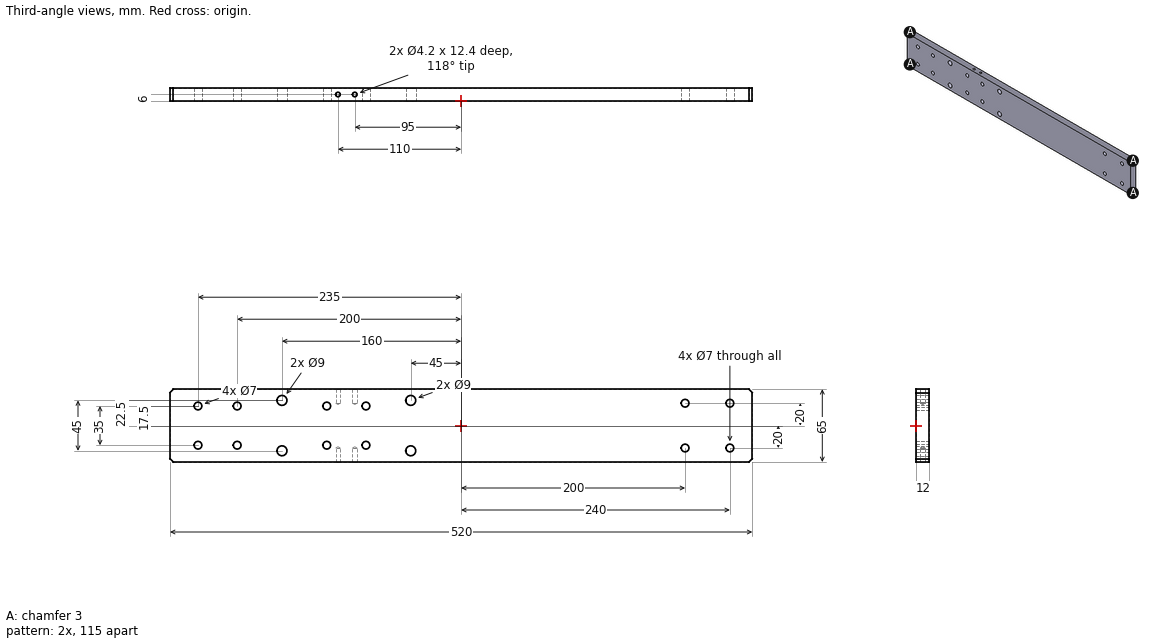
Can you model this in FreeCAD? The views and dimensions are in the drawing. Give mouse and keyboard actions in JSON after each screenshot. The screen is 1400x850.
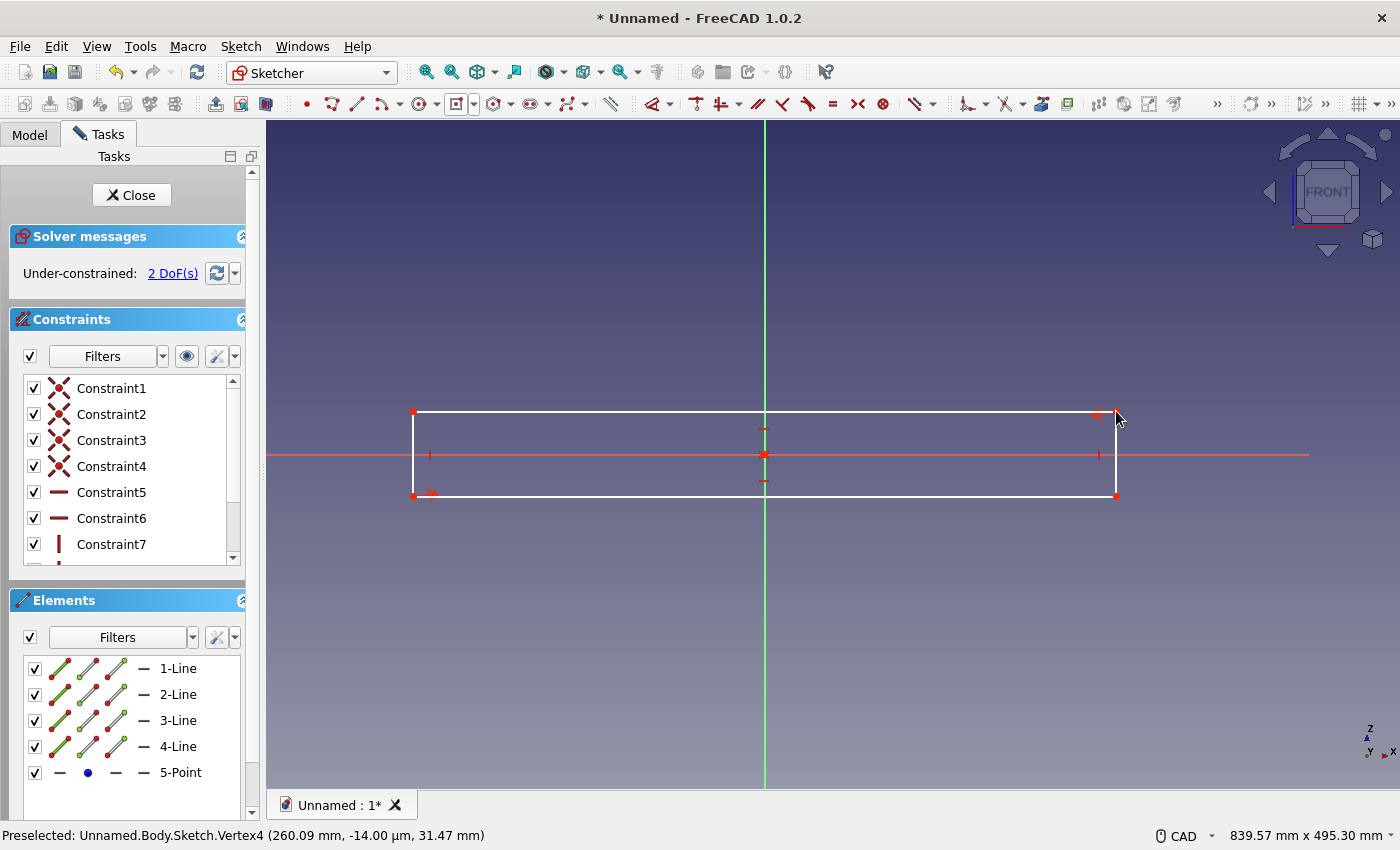
{"action": "left_click", "coordinate": [1116, 471]}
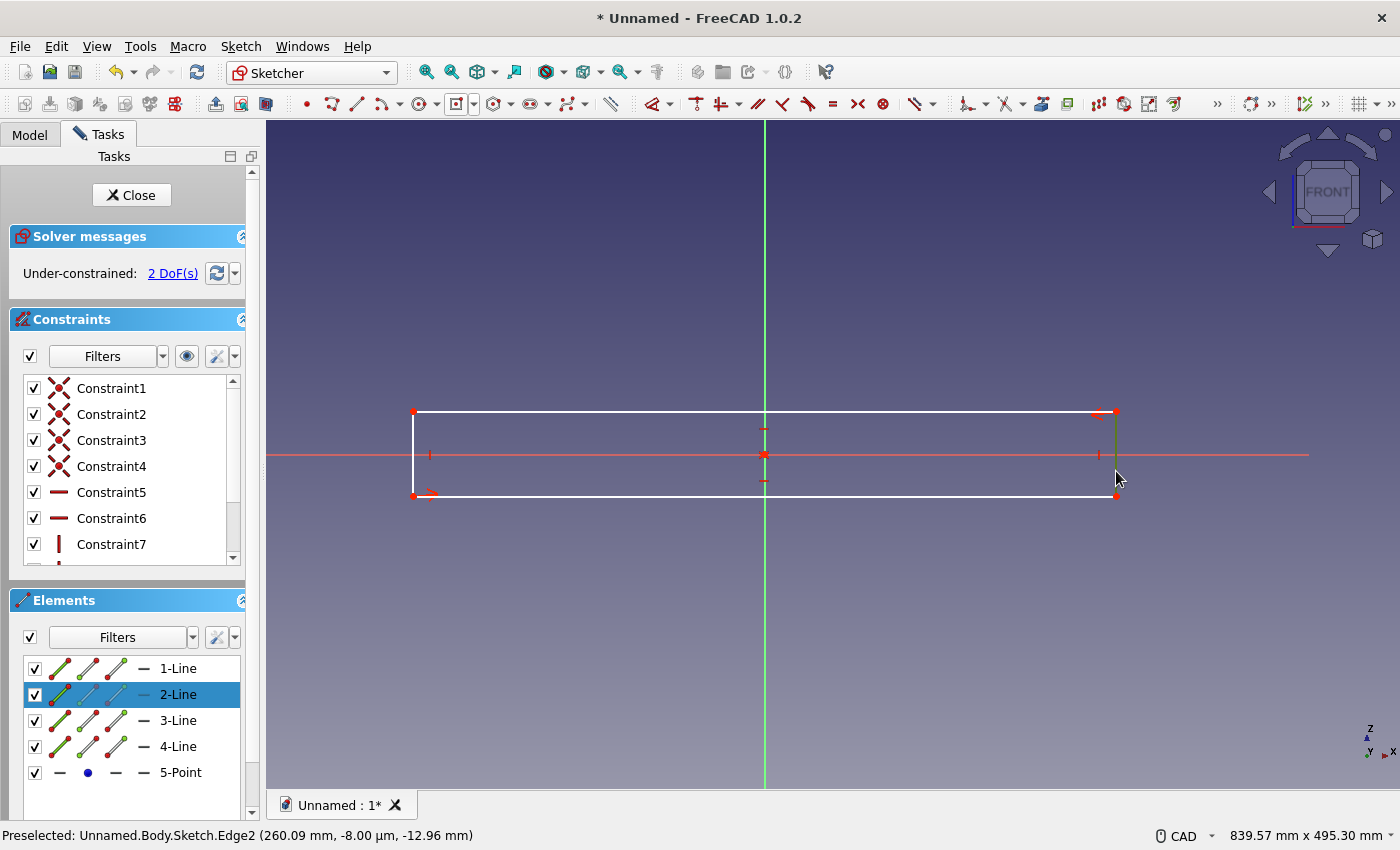
{"action": "left_click", "coordinate": [670, 104]}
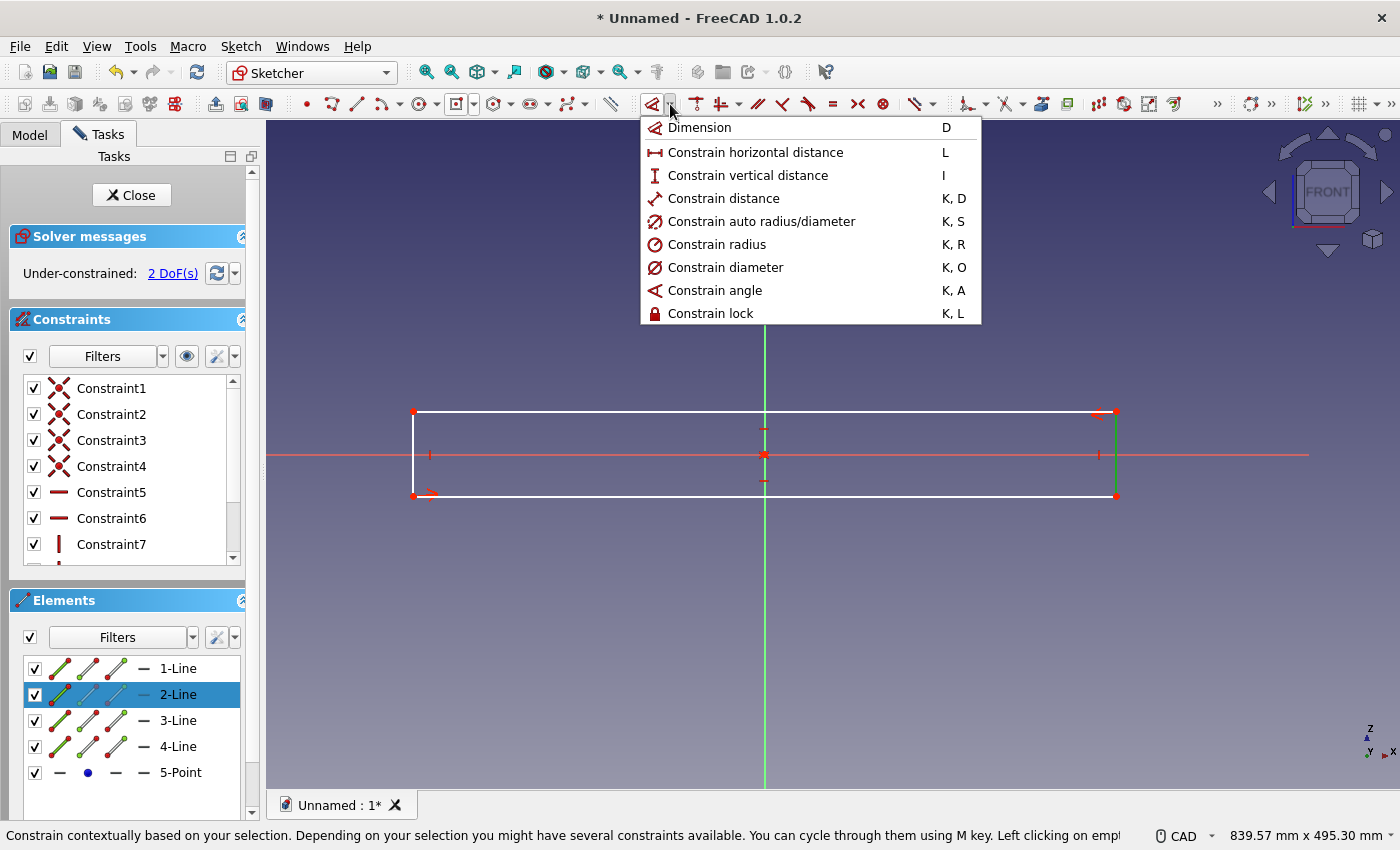
{"action": "left_click", "coordinate": [811, 176]}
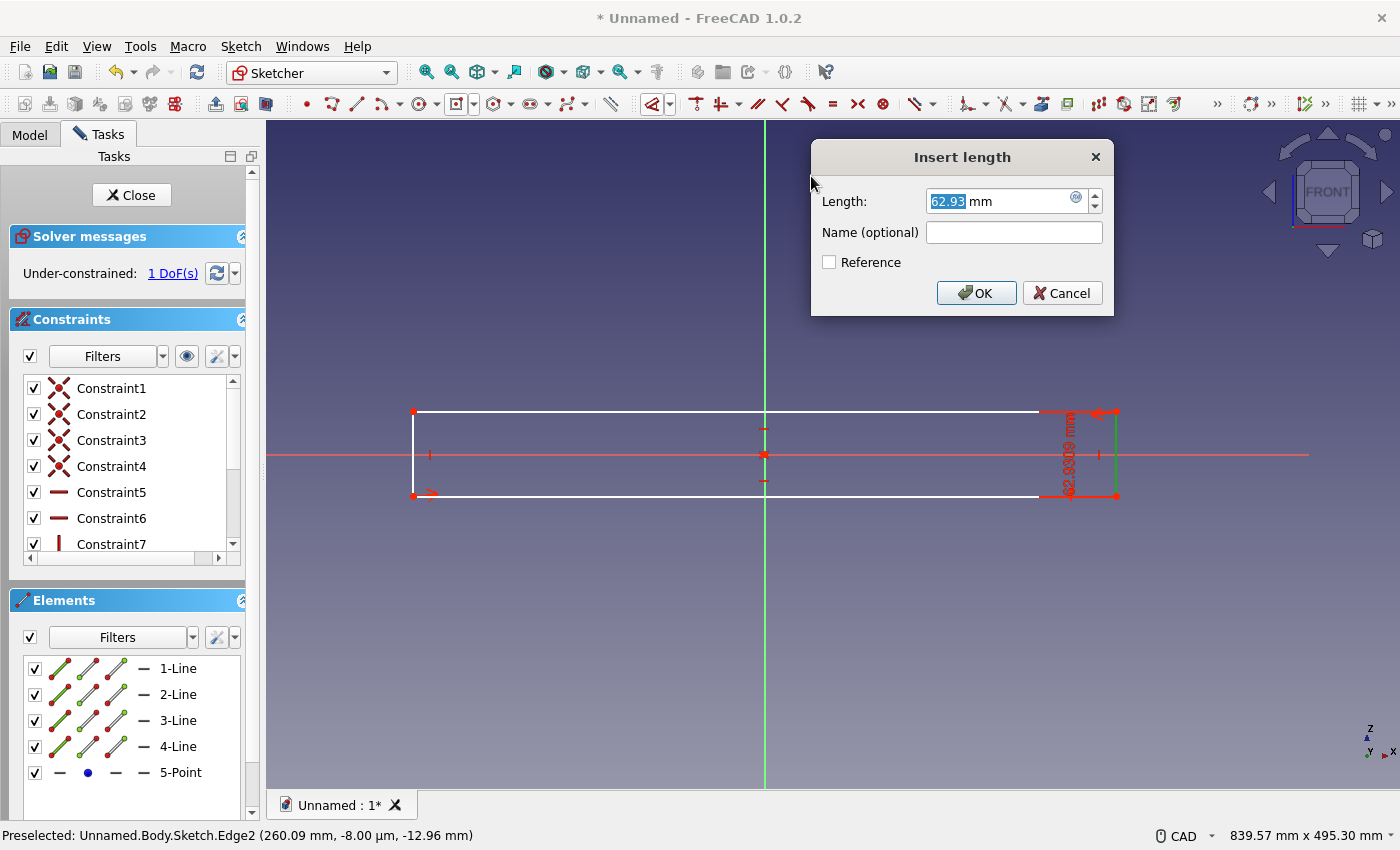
{"action": "type", "text": "65"}
{"action": "key", "text": "Return"}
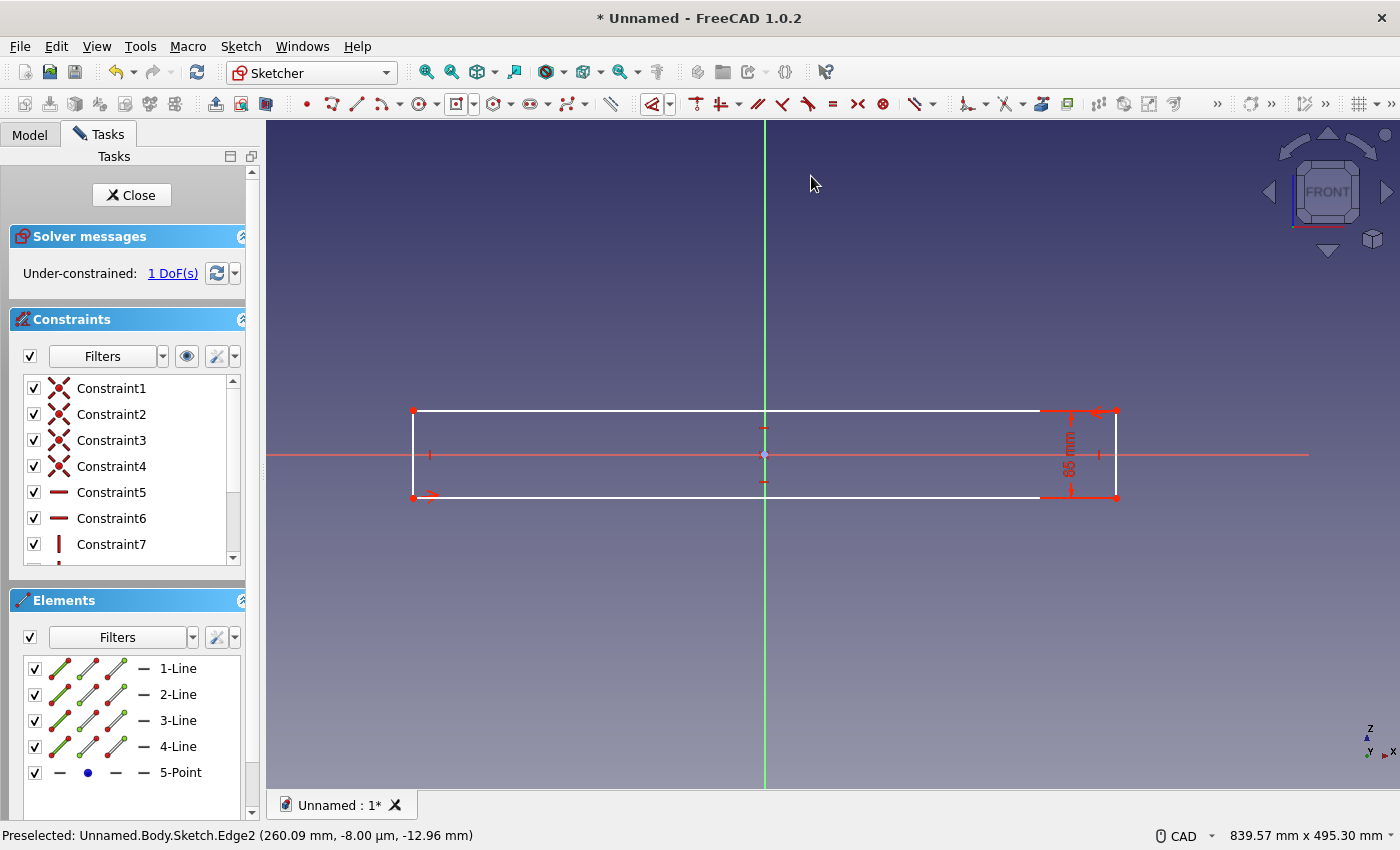
{"action": "left_click", "coordinate": [624, 498]}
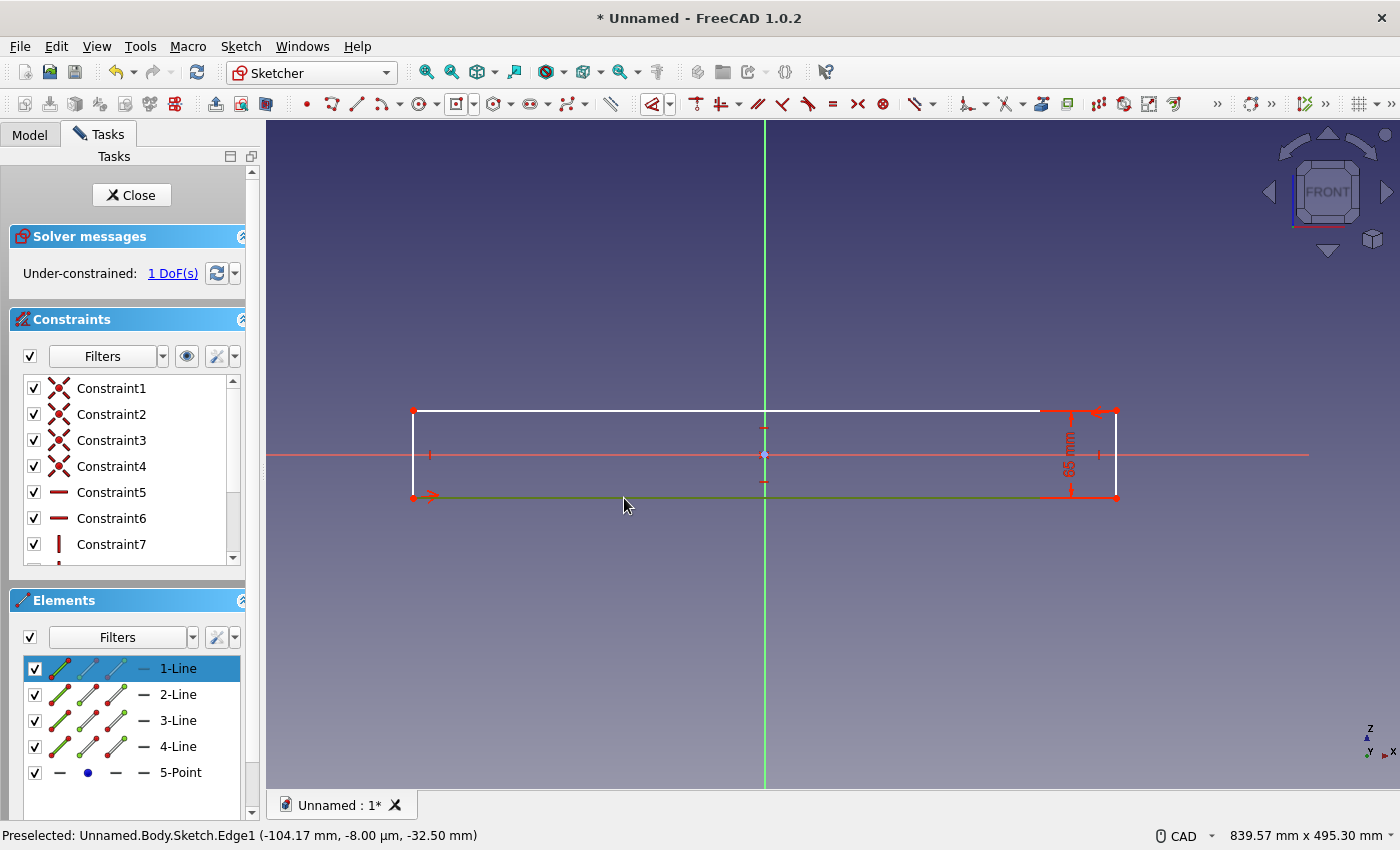
{"action": "key", "text": "l"}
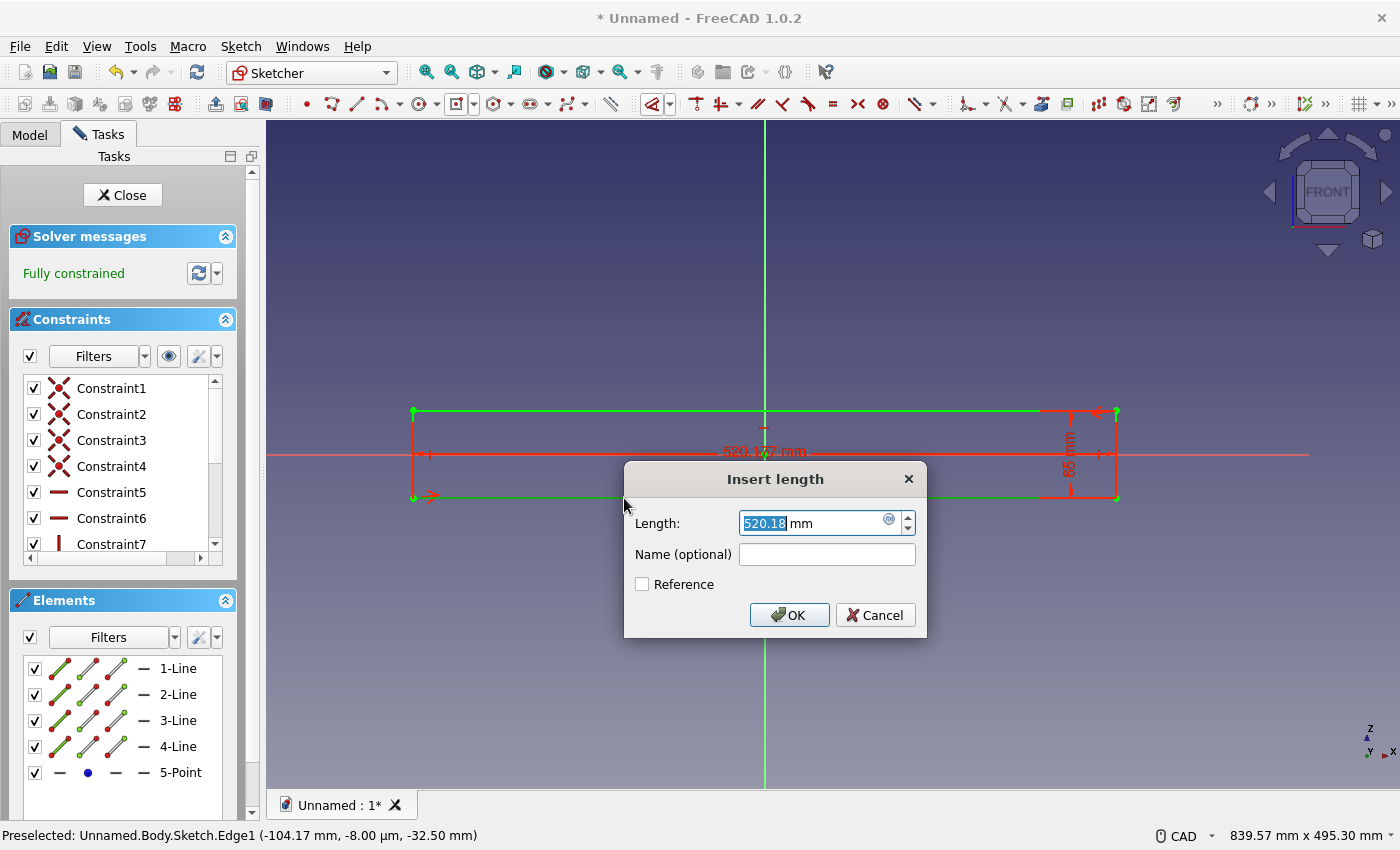
{"action": "type", "text": "520"}
{"action": "key", "text": "Return"}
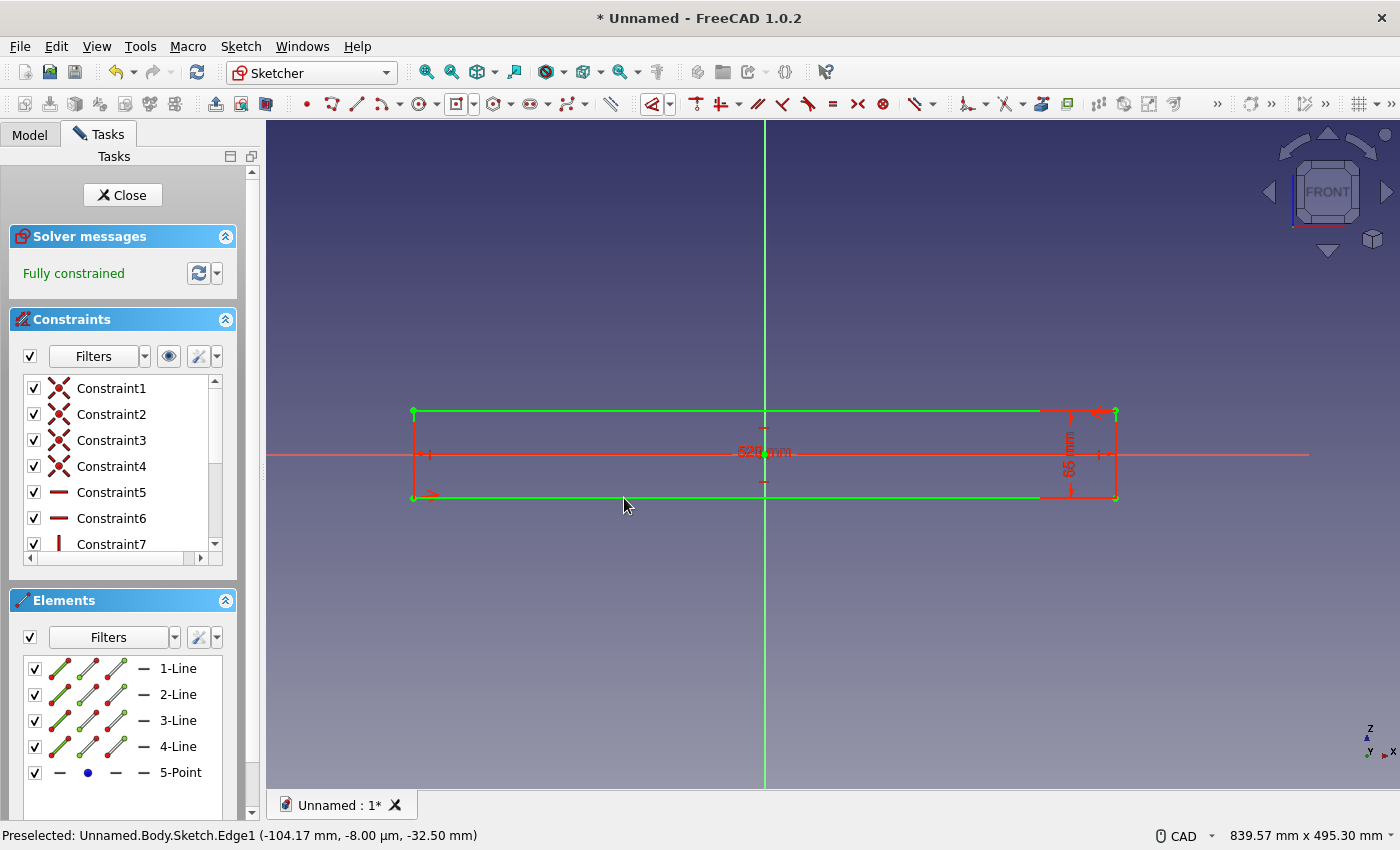
{"action": "left_click", "coordinate": [123, 195]}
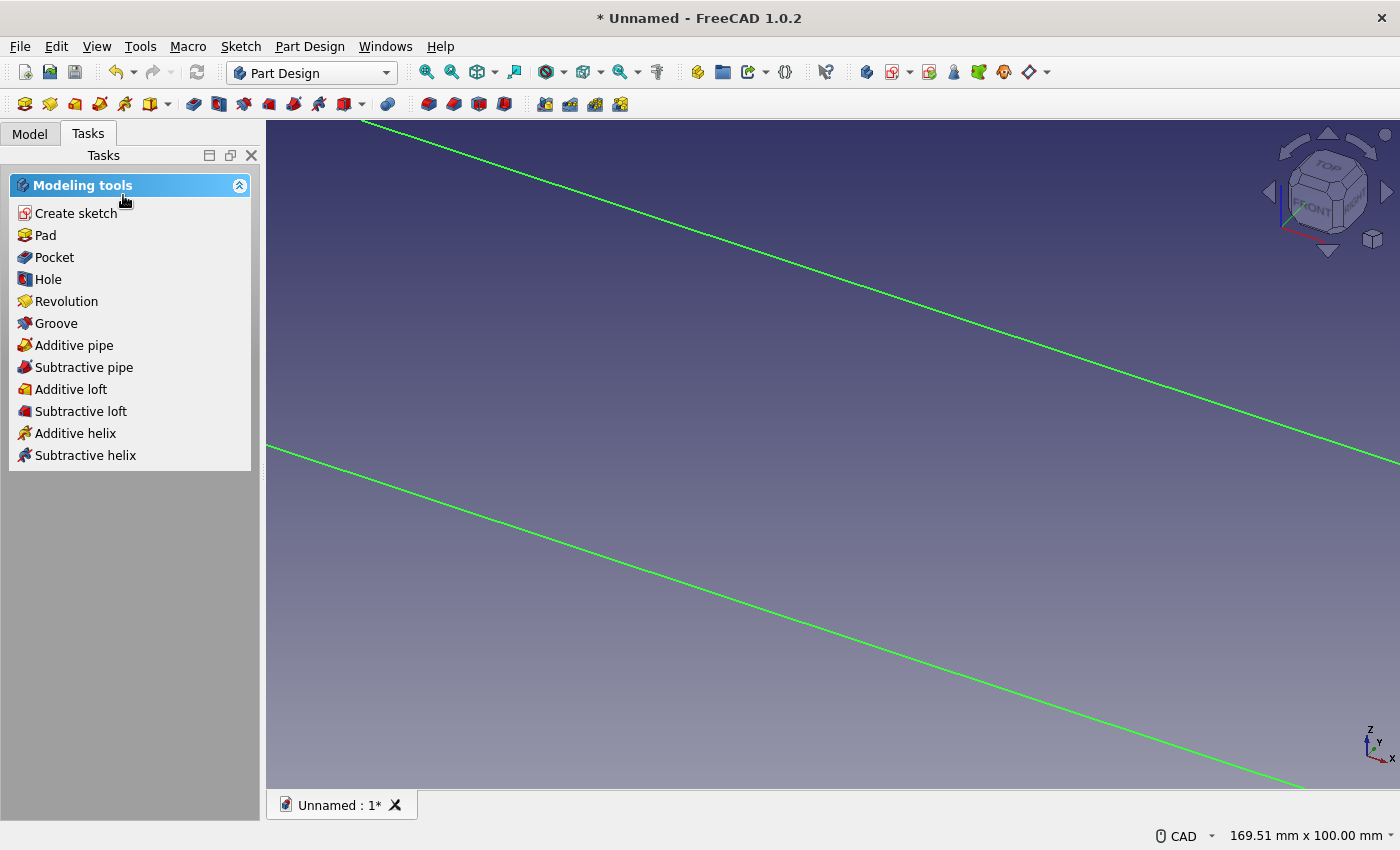
{"action": "left_click", "coordinate": [25, 104]}